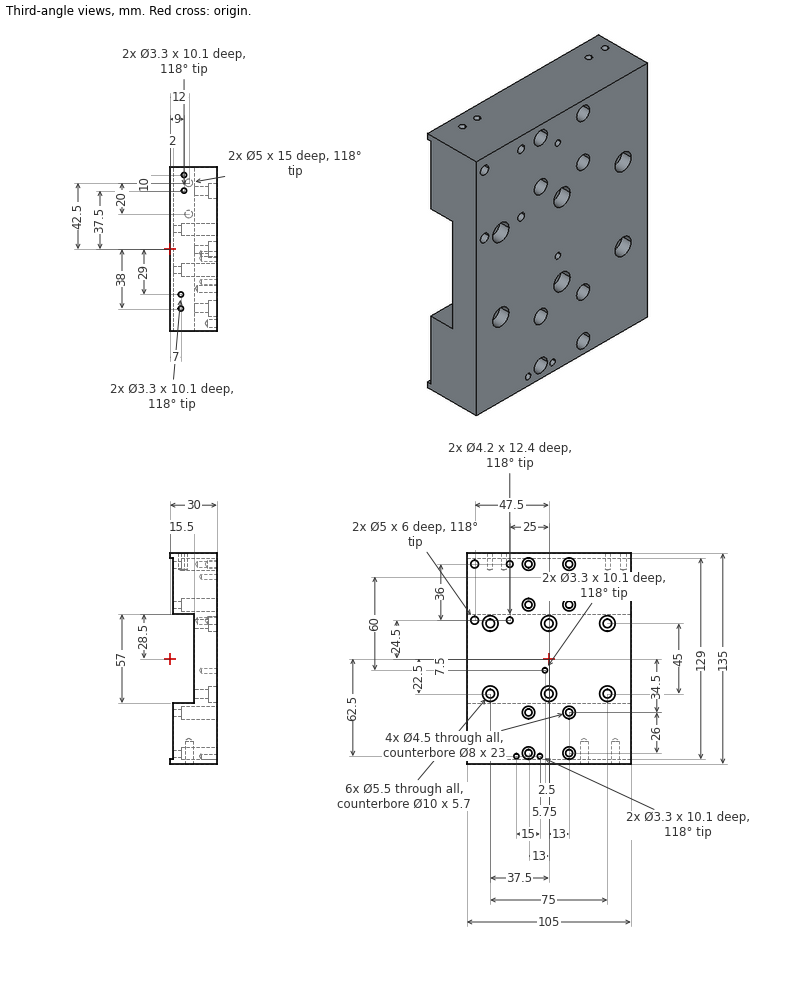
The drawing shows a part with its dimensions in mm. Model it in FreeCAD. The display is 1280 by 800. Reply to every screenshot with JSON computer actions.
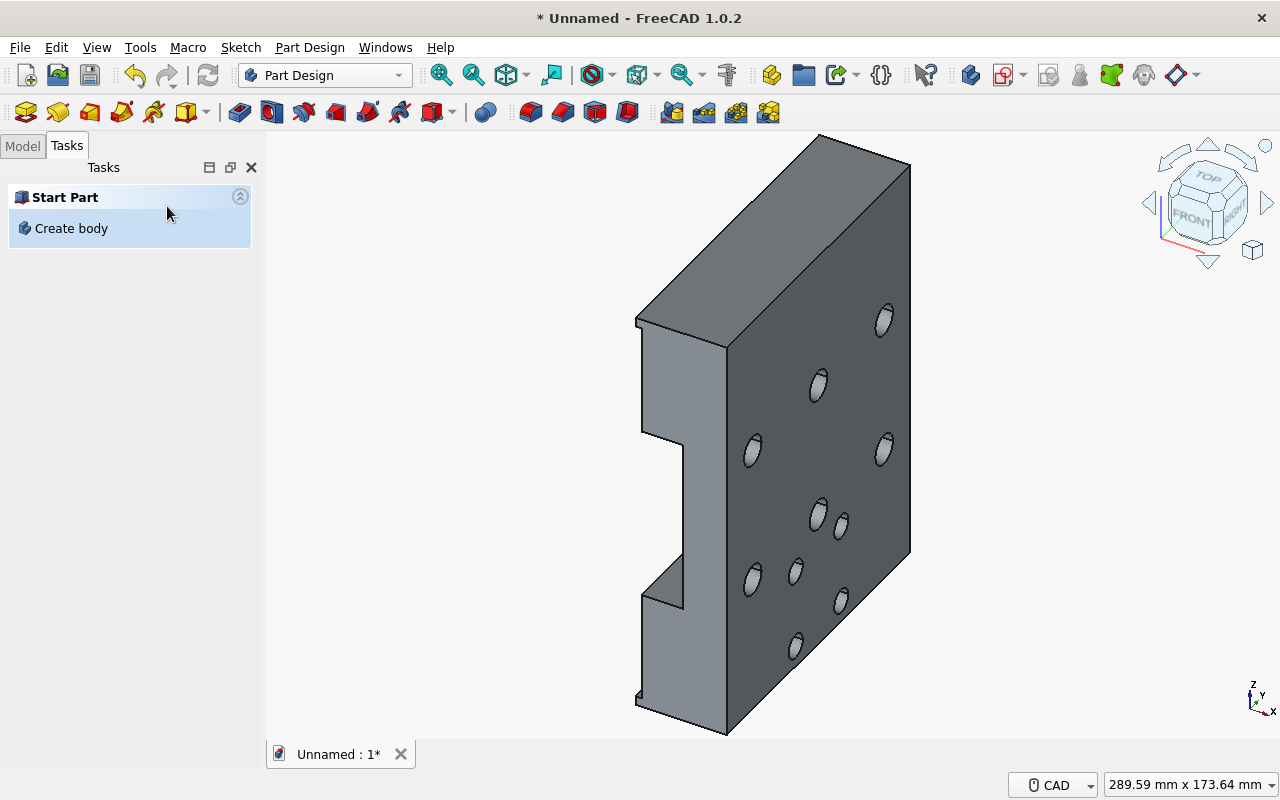
{"action": "left_click", "coordinate": [23, 145]}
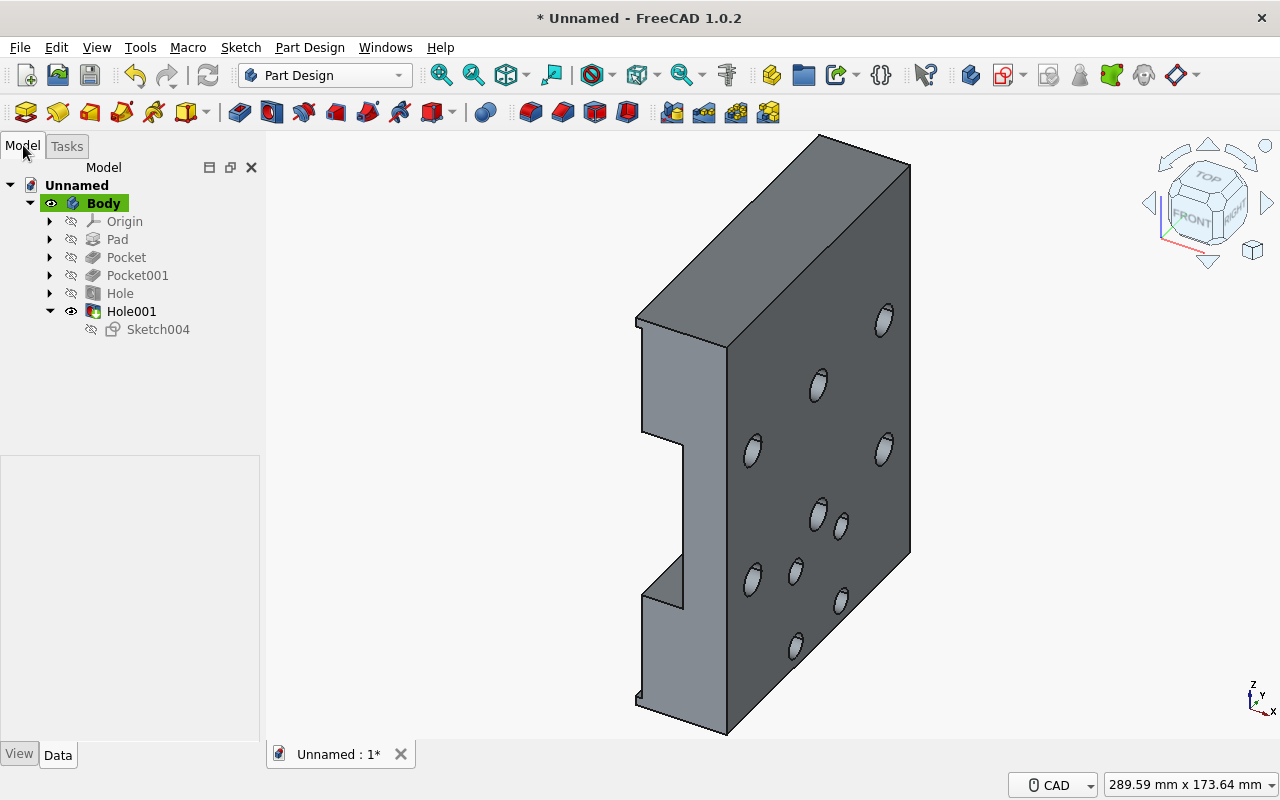
{"action": "left_click", "coordinate": [116, 311]}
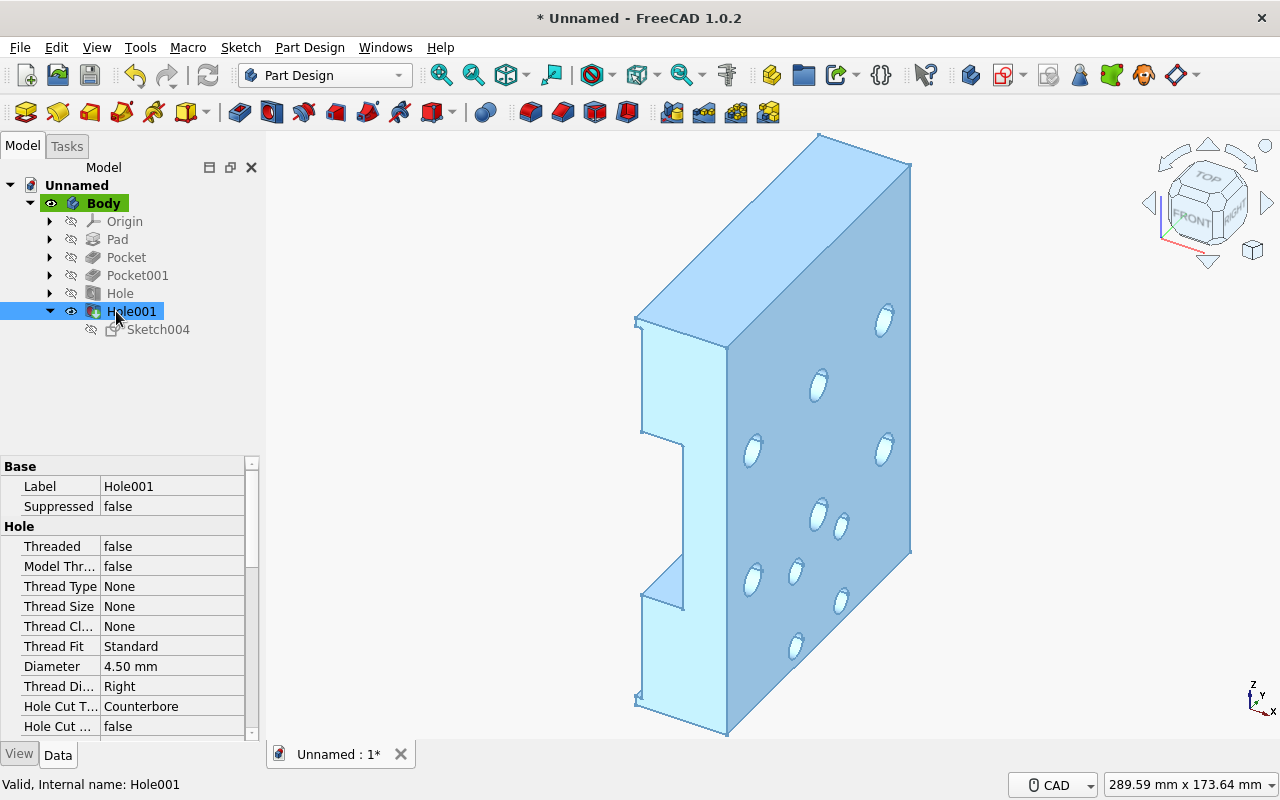
{"action": "left_click", "coordinate": [672, 112]}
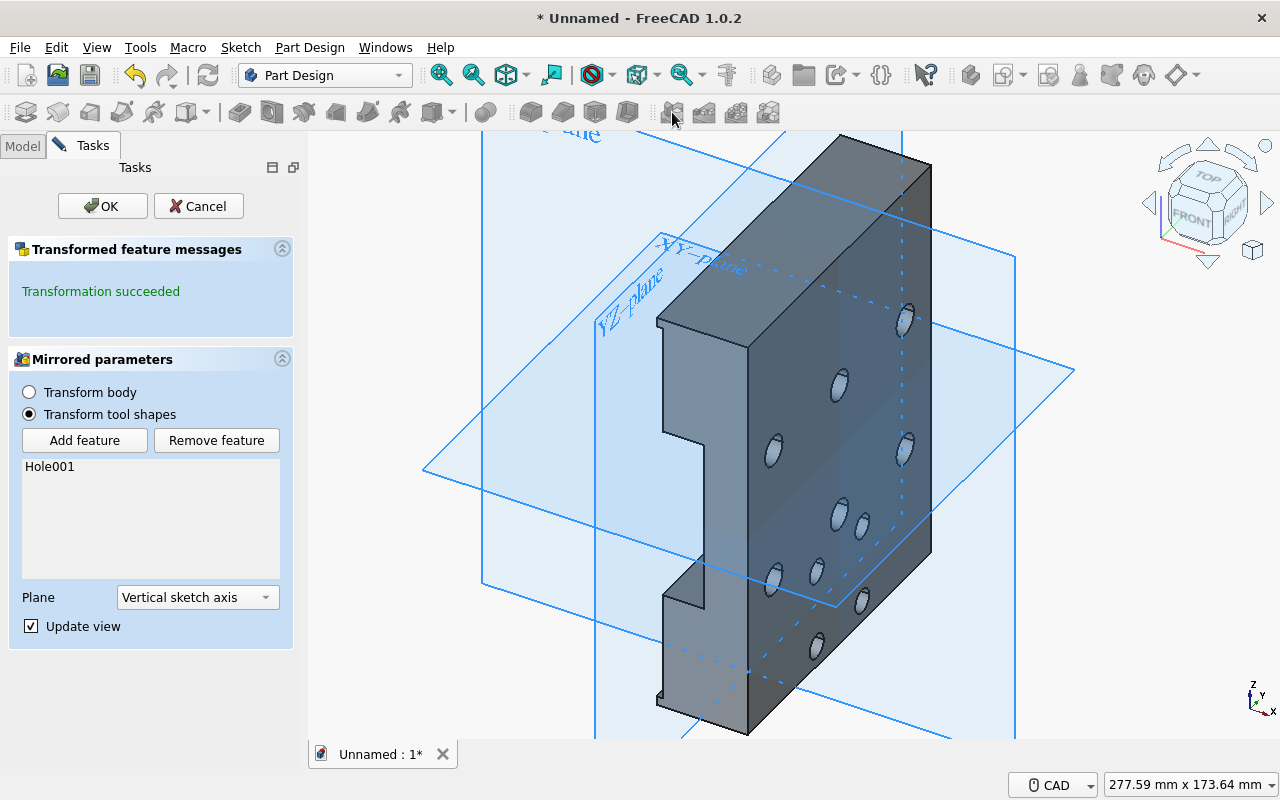
{"action": "left_click", "coordinate": [198, 598]}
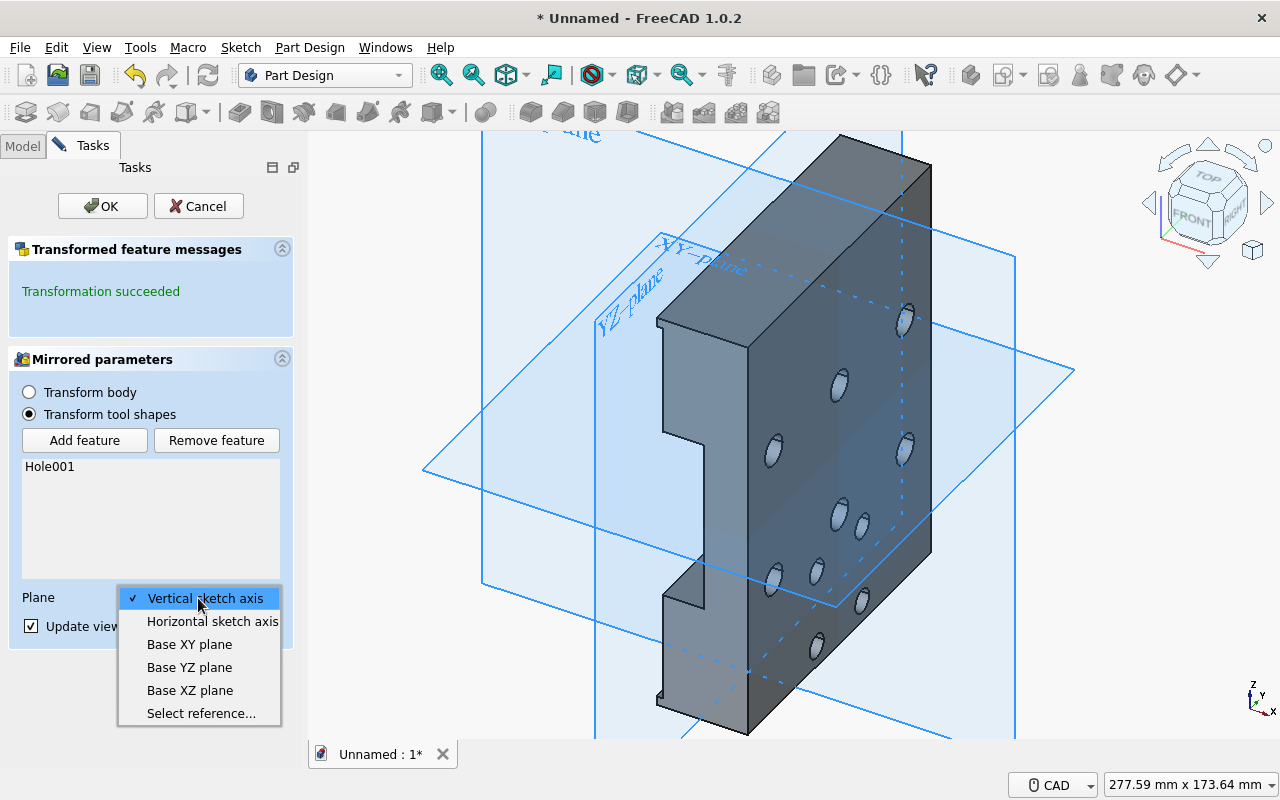
{"action": "left_click", "coordinate": [198, 644]}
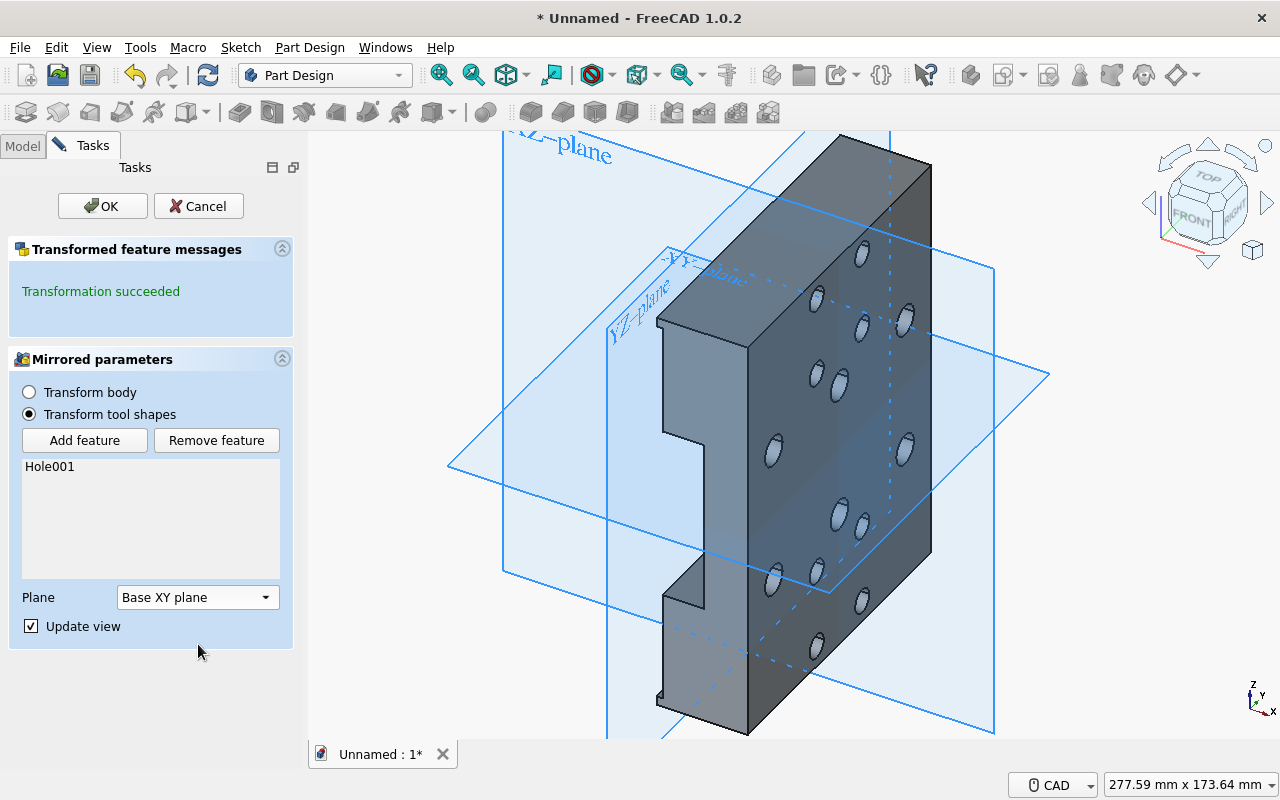
{"action": "left_click", "coordinate": [103, 206]}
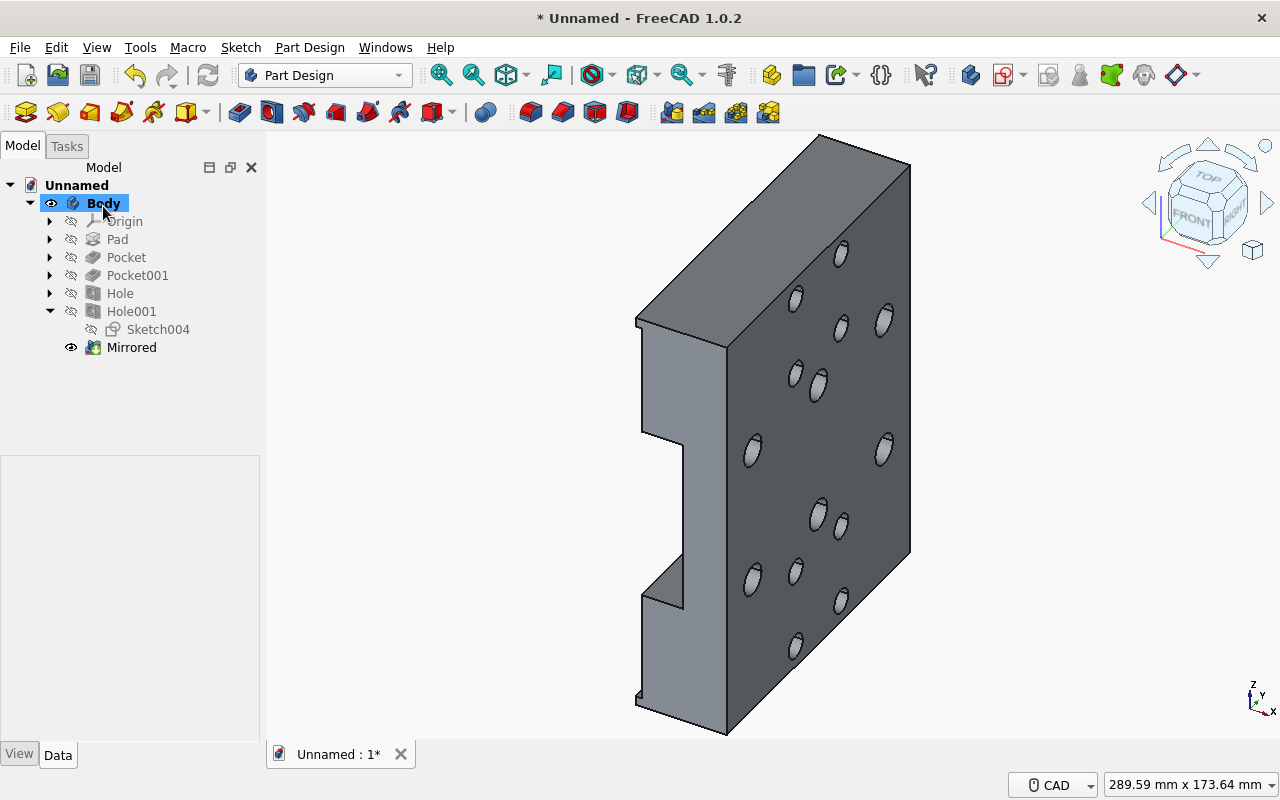
{"action": "left_click", "coordinate": [845, 423]}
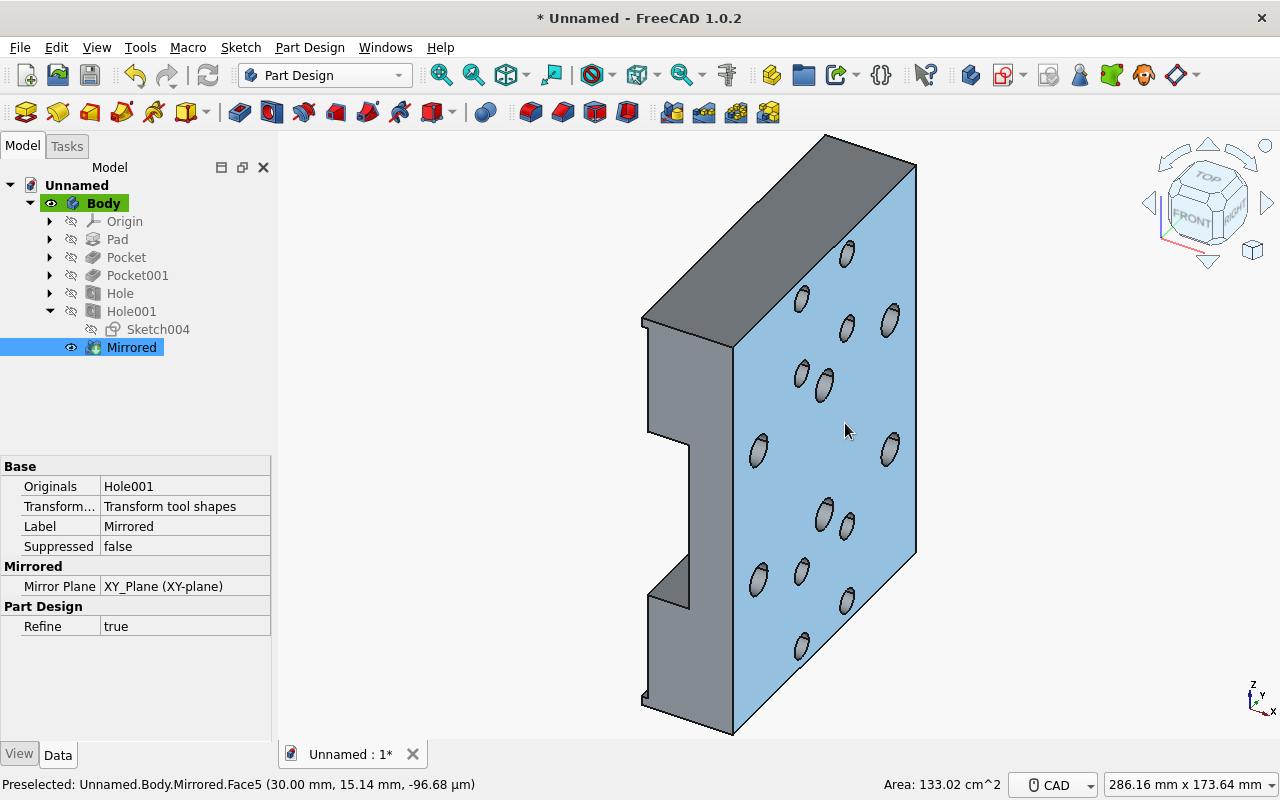
{"action": "left_click", "coordinate": [1004, 76]}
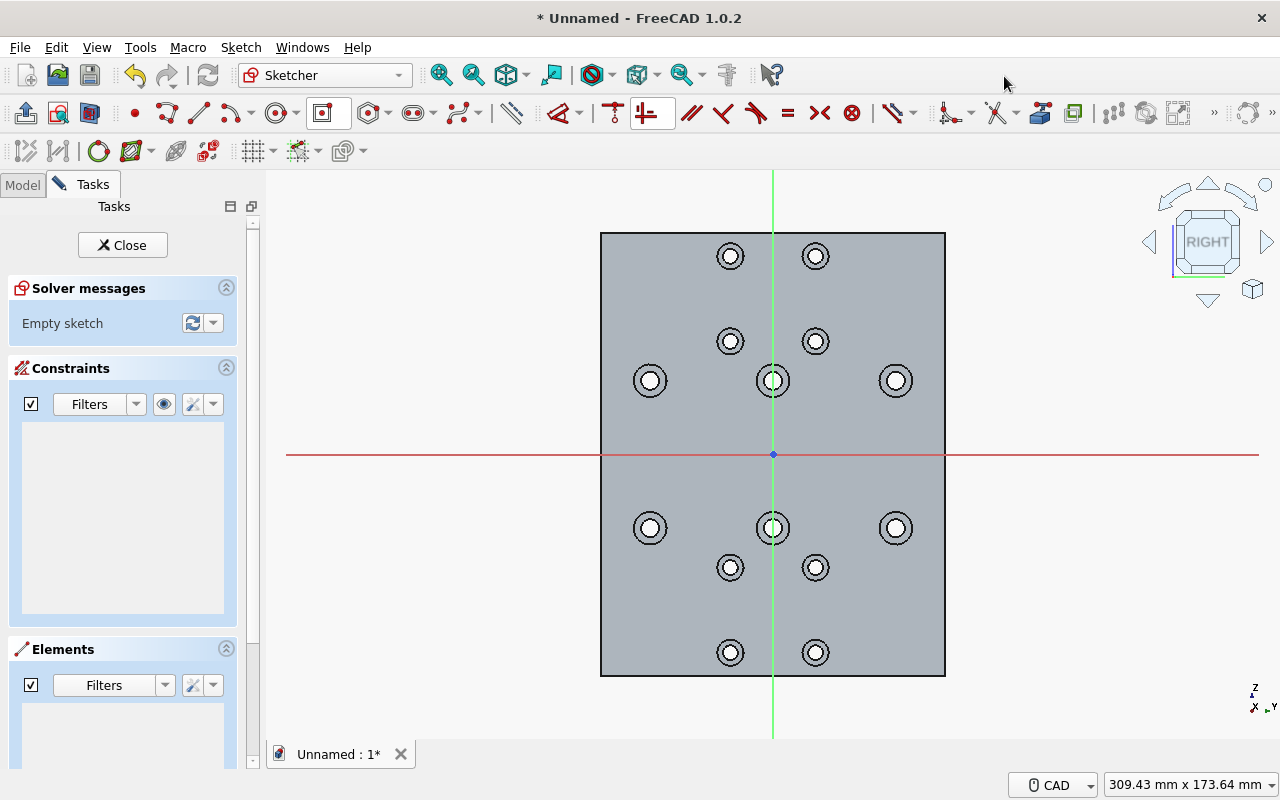
{"action": "scroll", "coordinate": [733, 685], "scroll_direction": "up", "scroll_amount": 11}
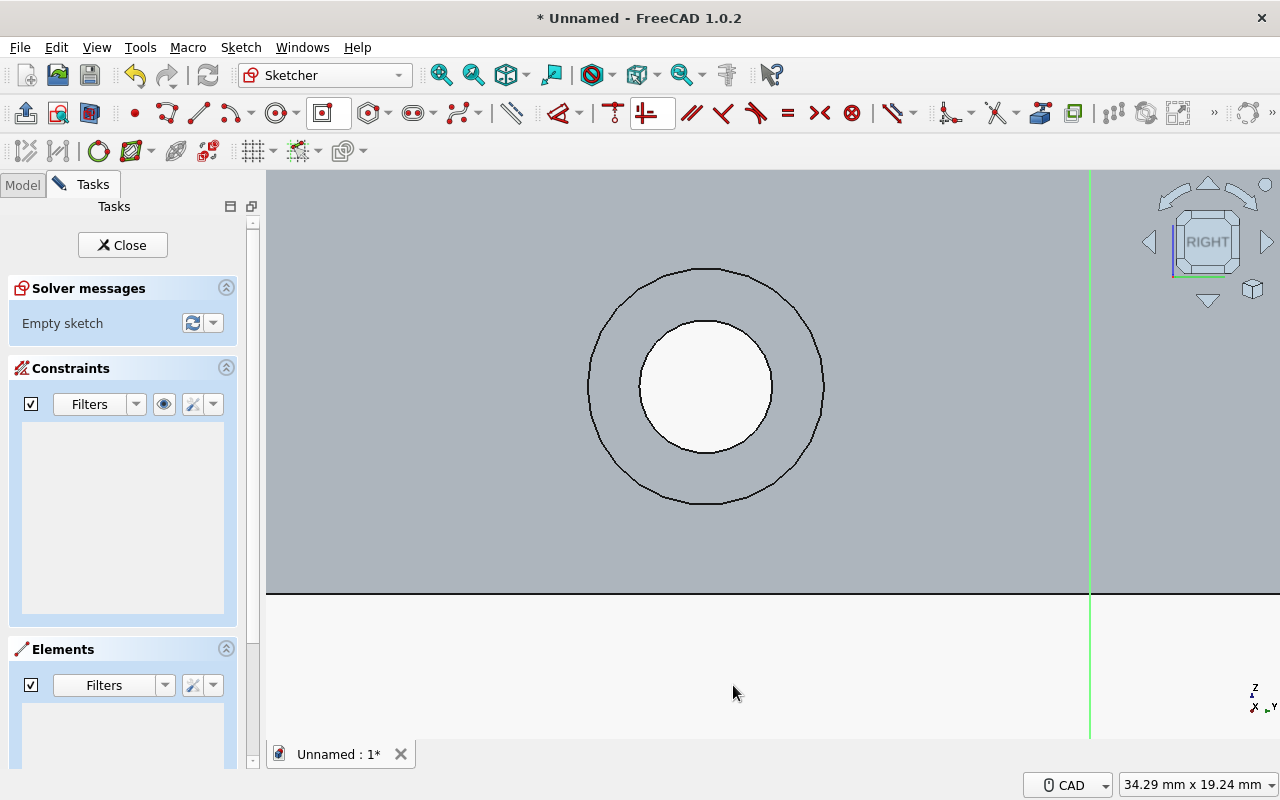
{"action": "left_click", "coordinate": [276, 114]}